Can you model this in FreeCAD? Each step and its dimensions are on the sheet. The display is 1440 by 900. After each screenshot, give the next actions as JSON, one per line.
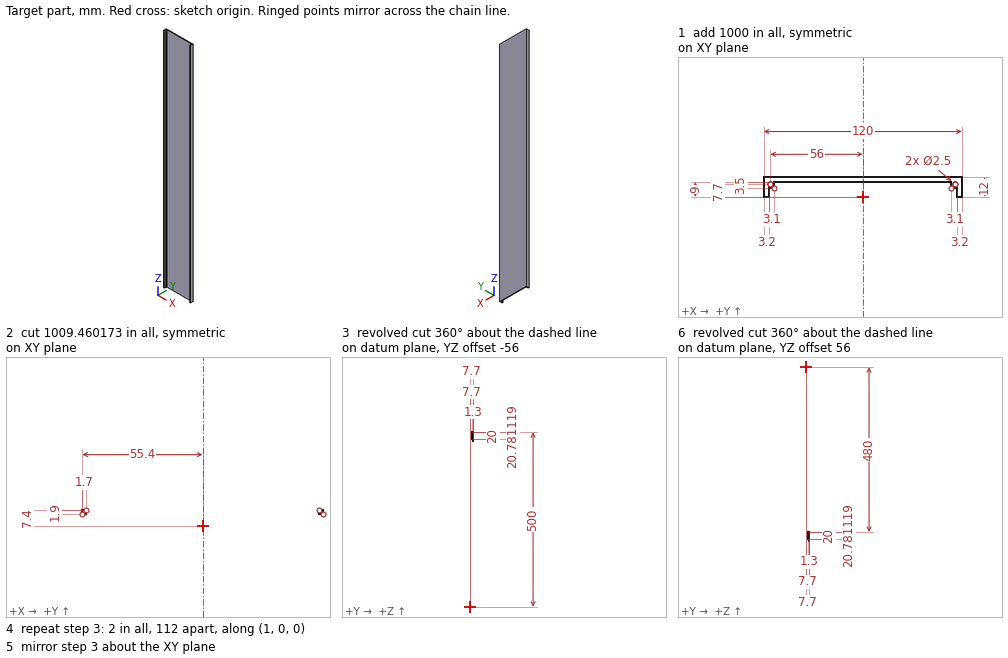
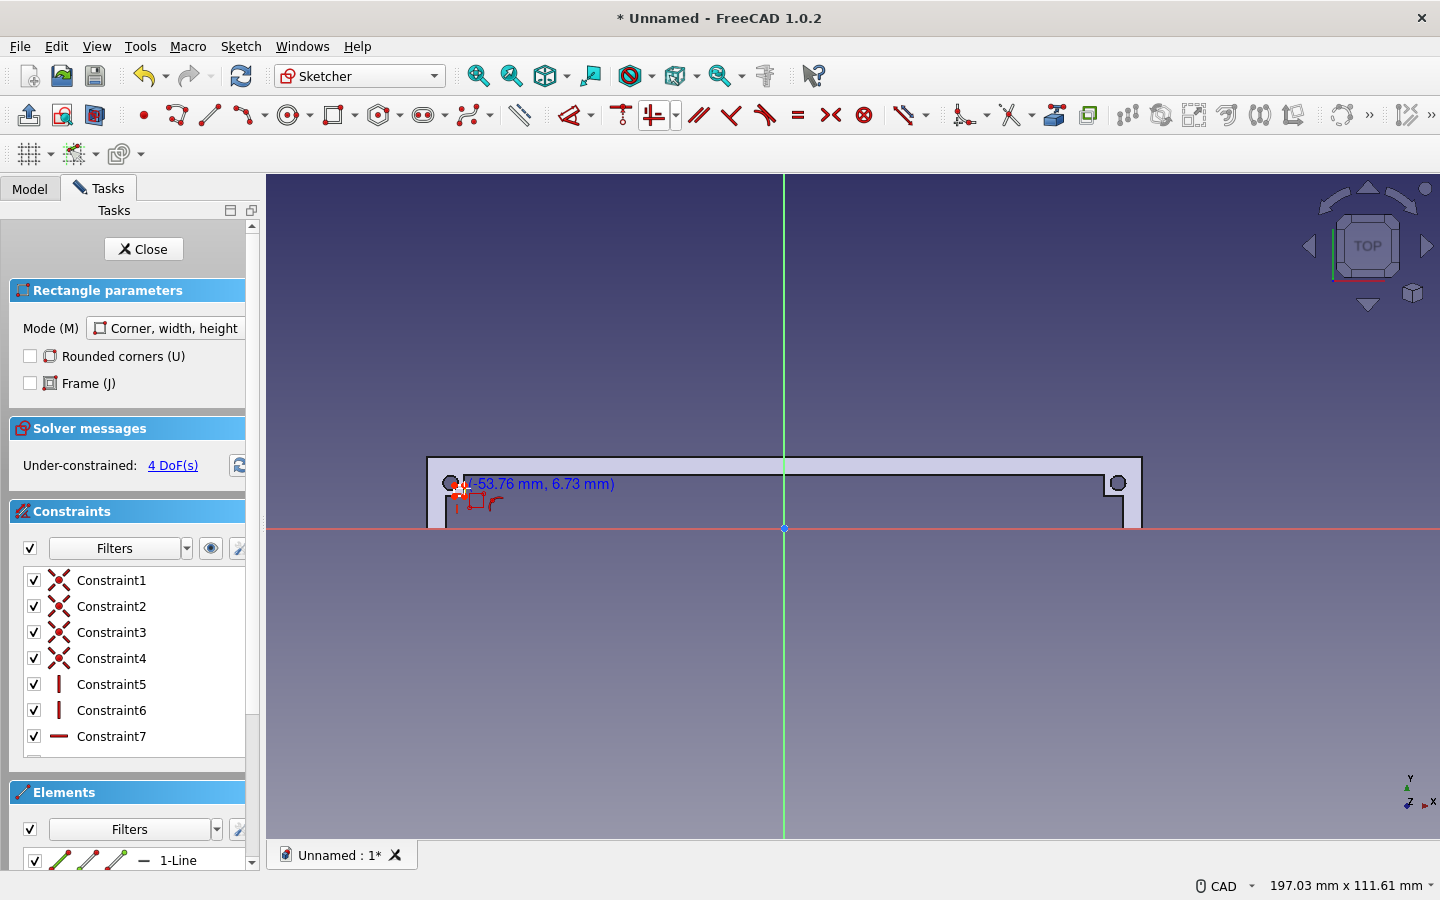
{"action": "scroll", "coordinate": [1104, 485], "scroll_direction": "up", "scroll_amount": 3}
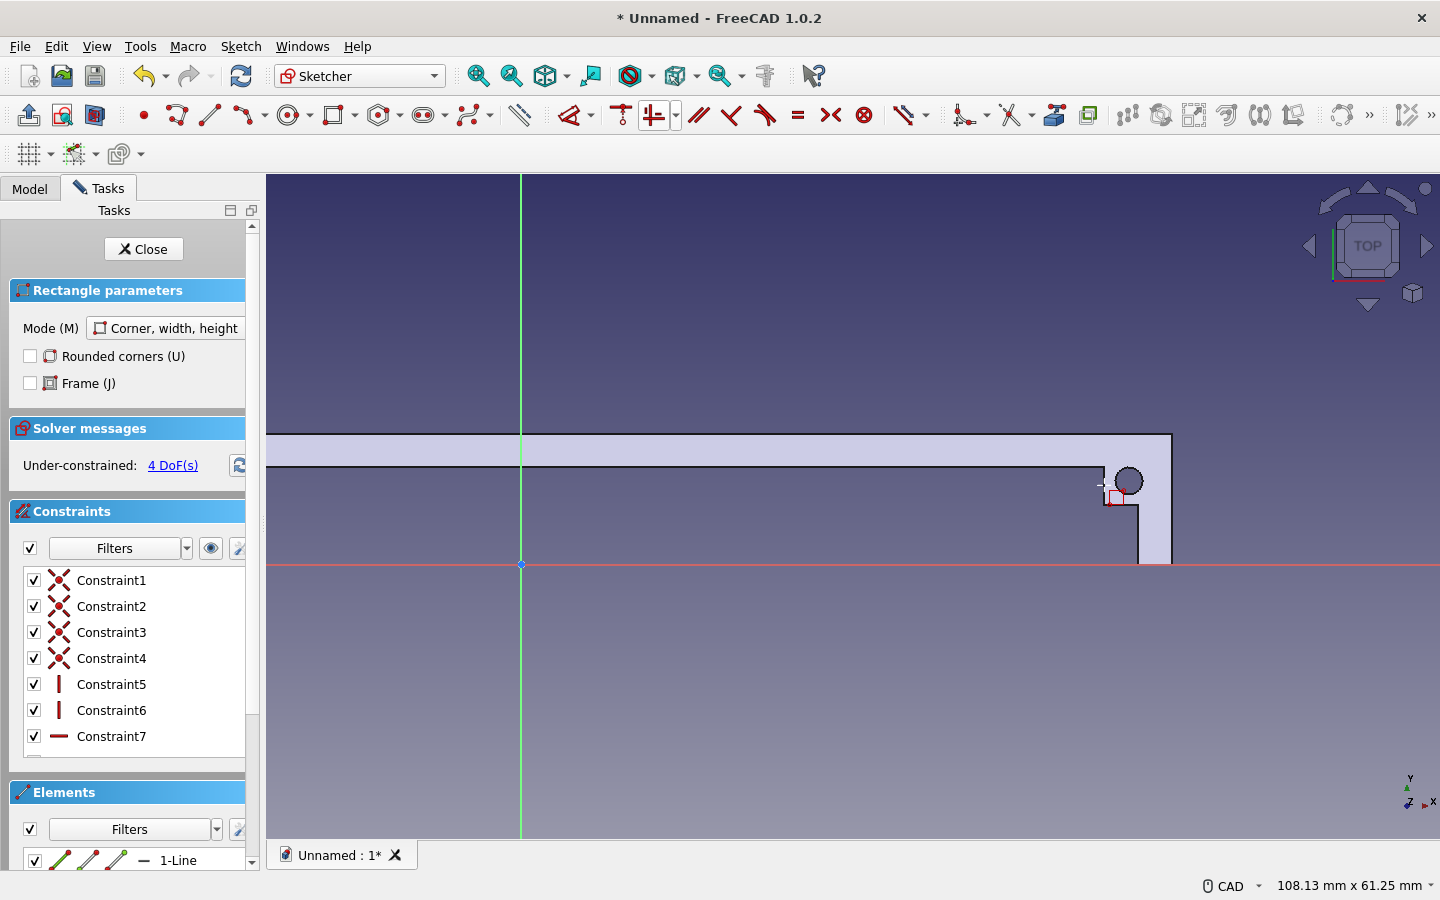
{"action": "left_click", "coordinate": [1104, 484]}
{"action": "left_click", "coordinate": [1122, 505]}
{"action": "key", "text": "Escape"}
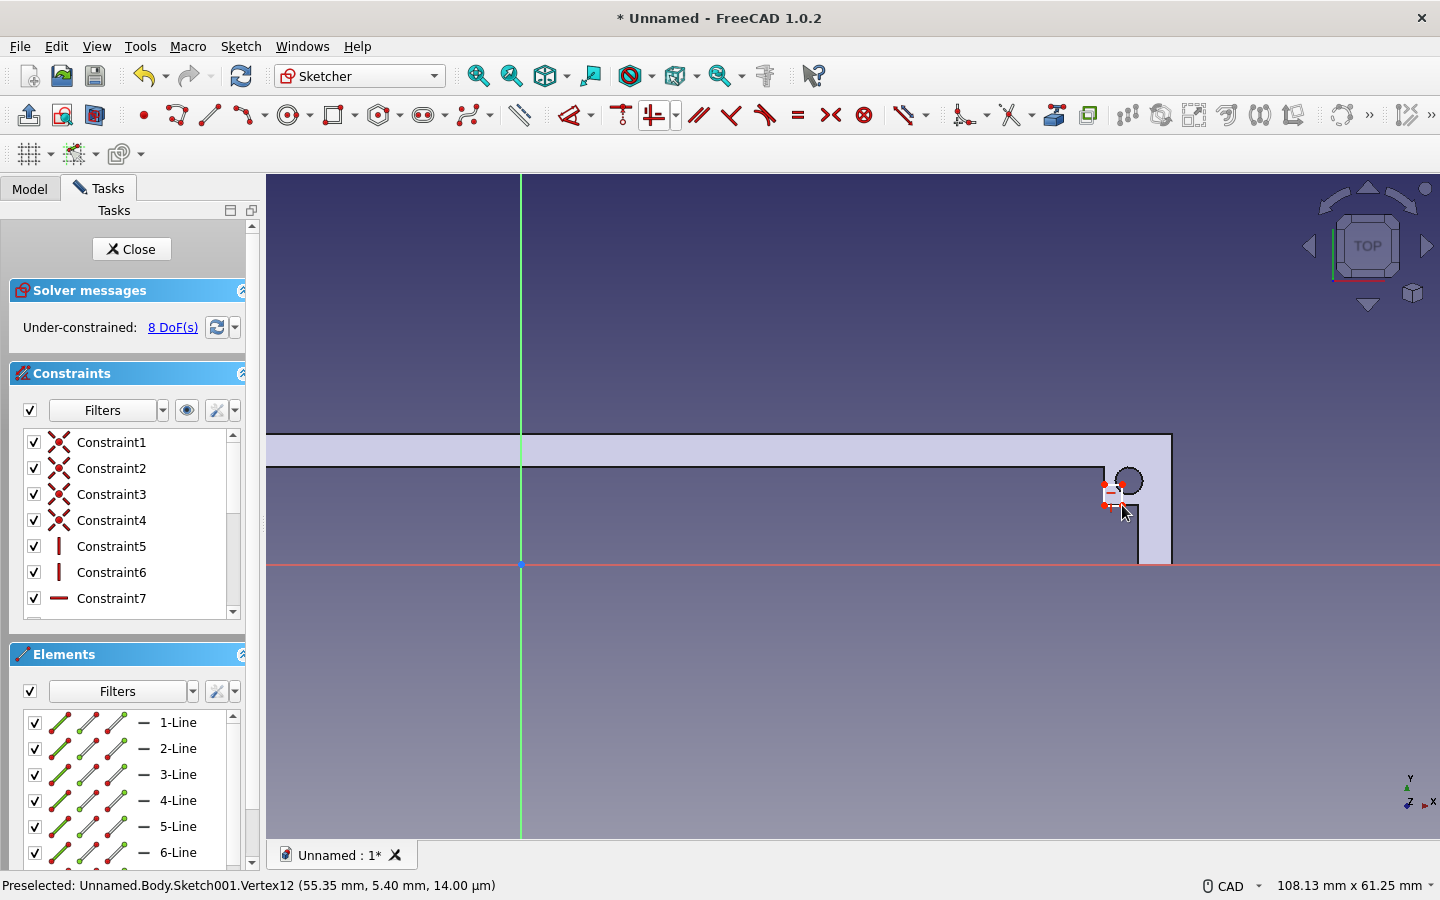
{"action": "scroll", "coordinate": [1105, 485], "scroll_direction": "down", "scroll_amount": 3}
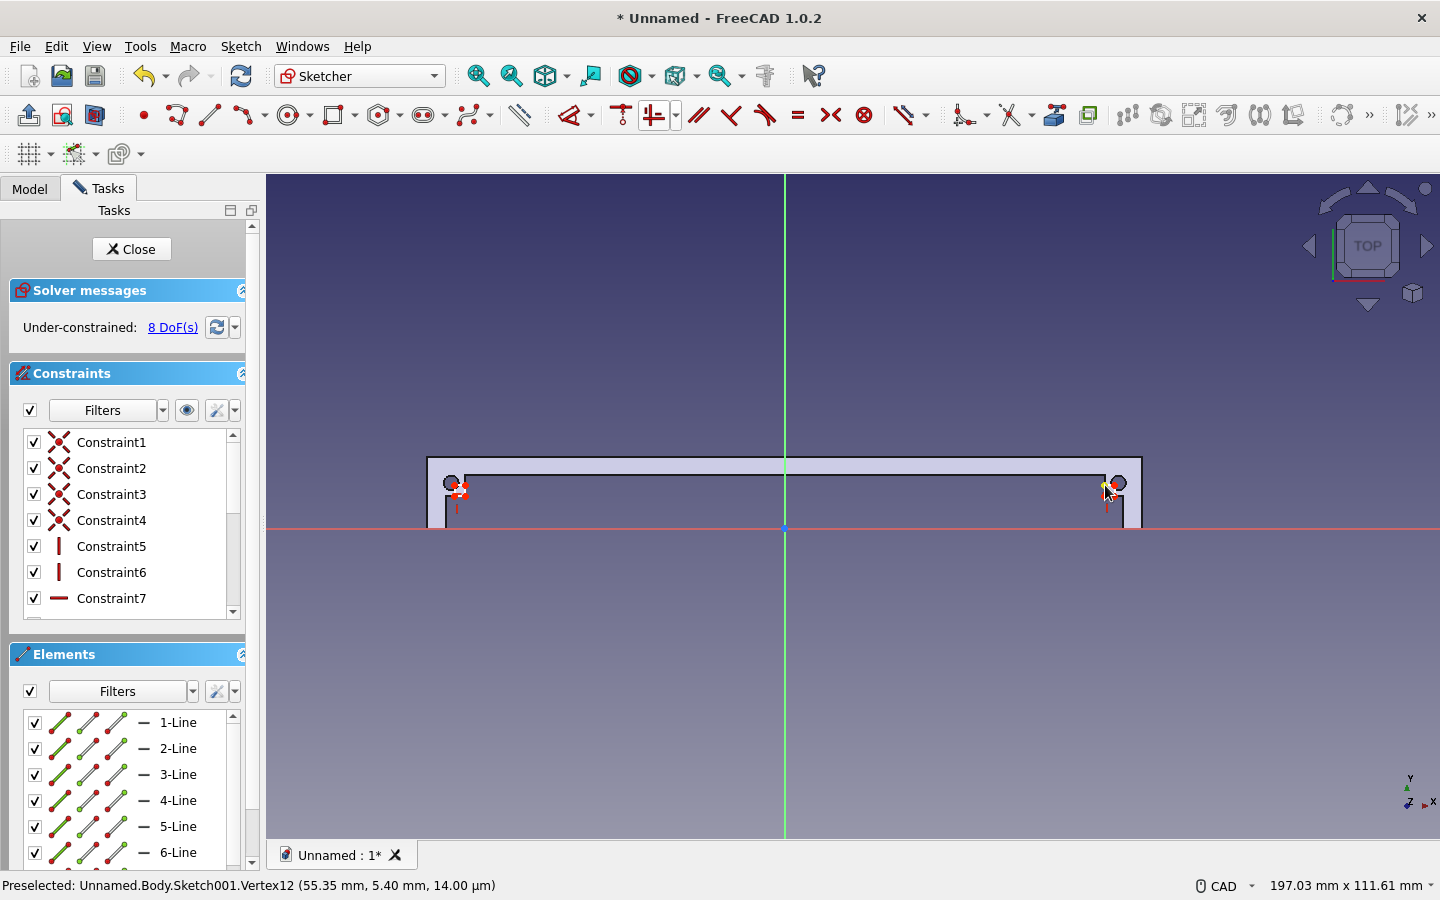
{"action": "left_click", "coordinate": [465, 485]}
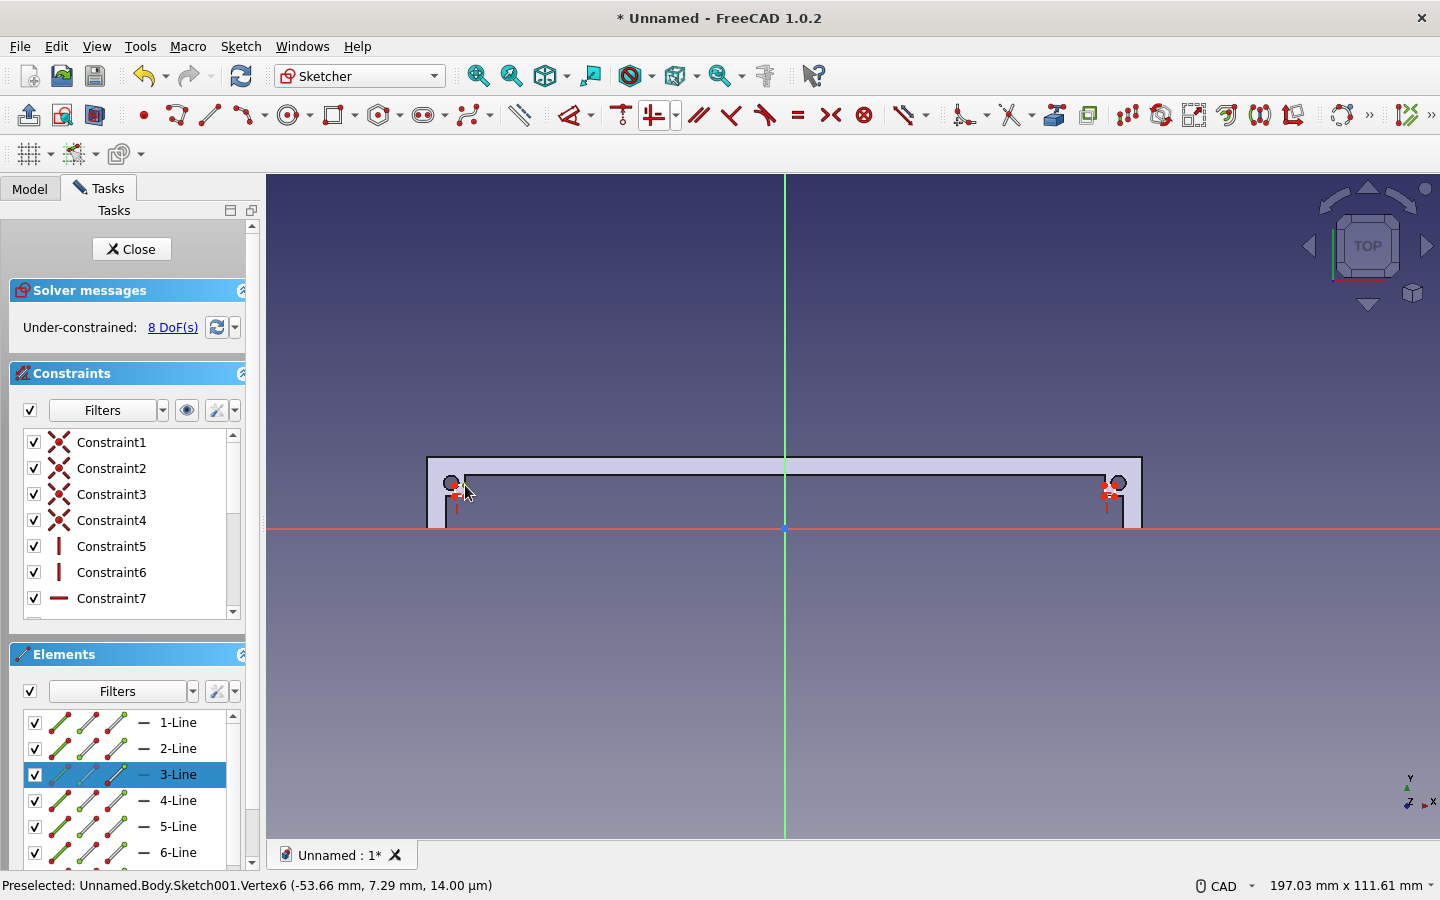
{"action": "scroll", "coordinate": [1105, 485], "scroll_direction": "up", "scroll_amount": 2}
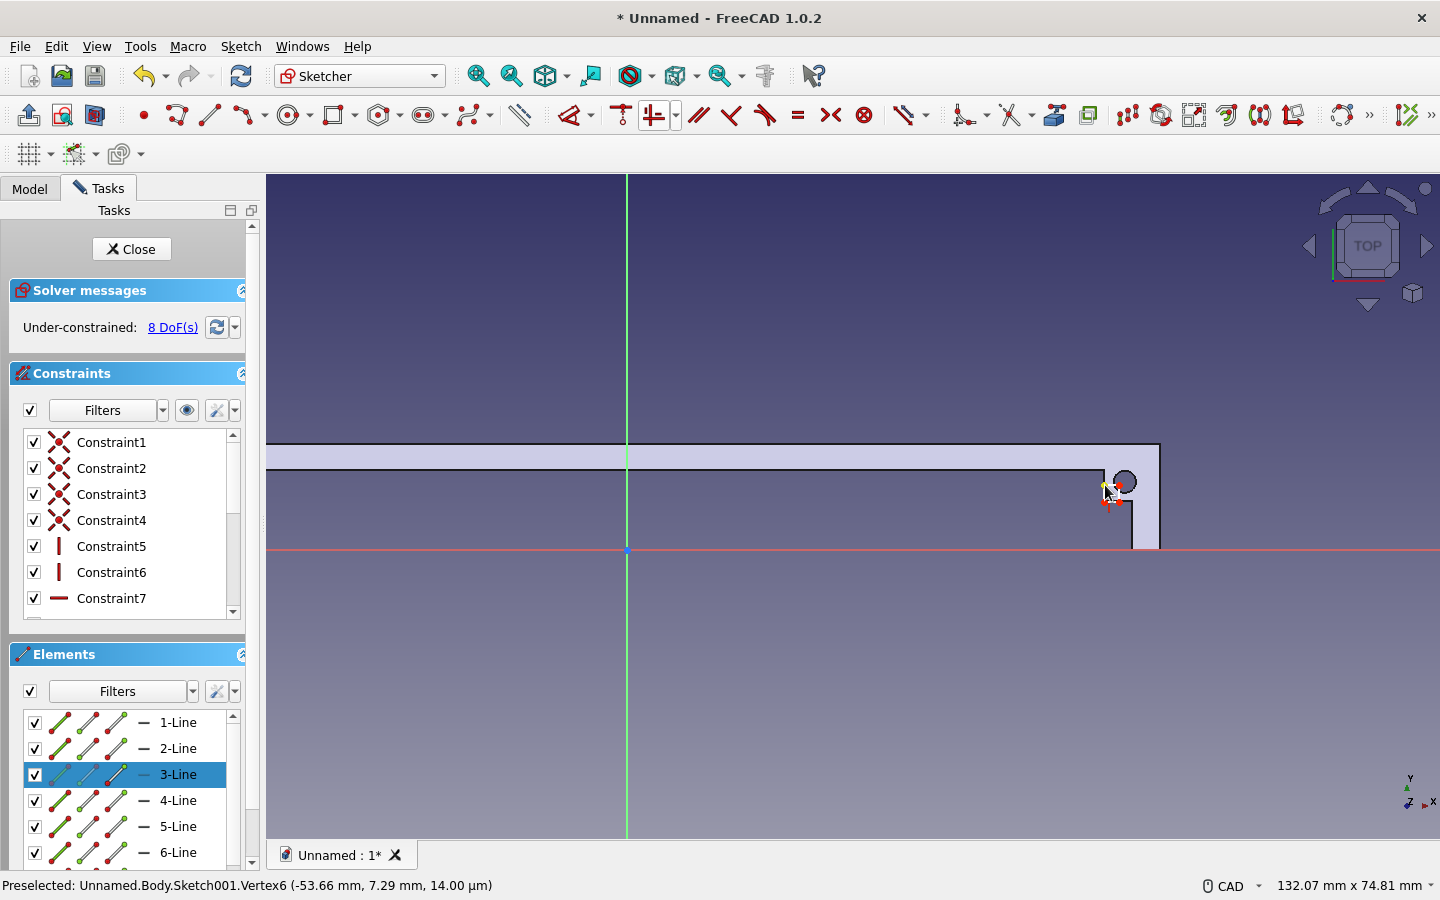
{"action": "left_click", "coordinate": [1104, 485]}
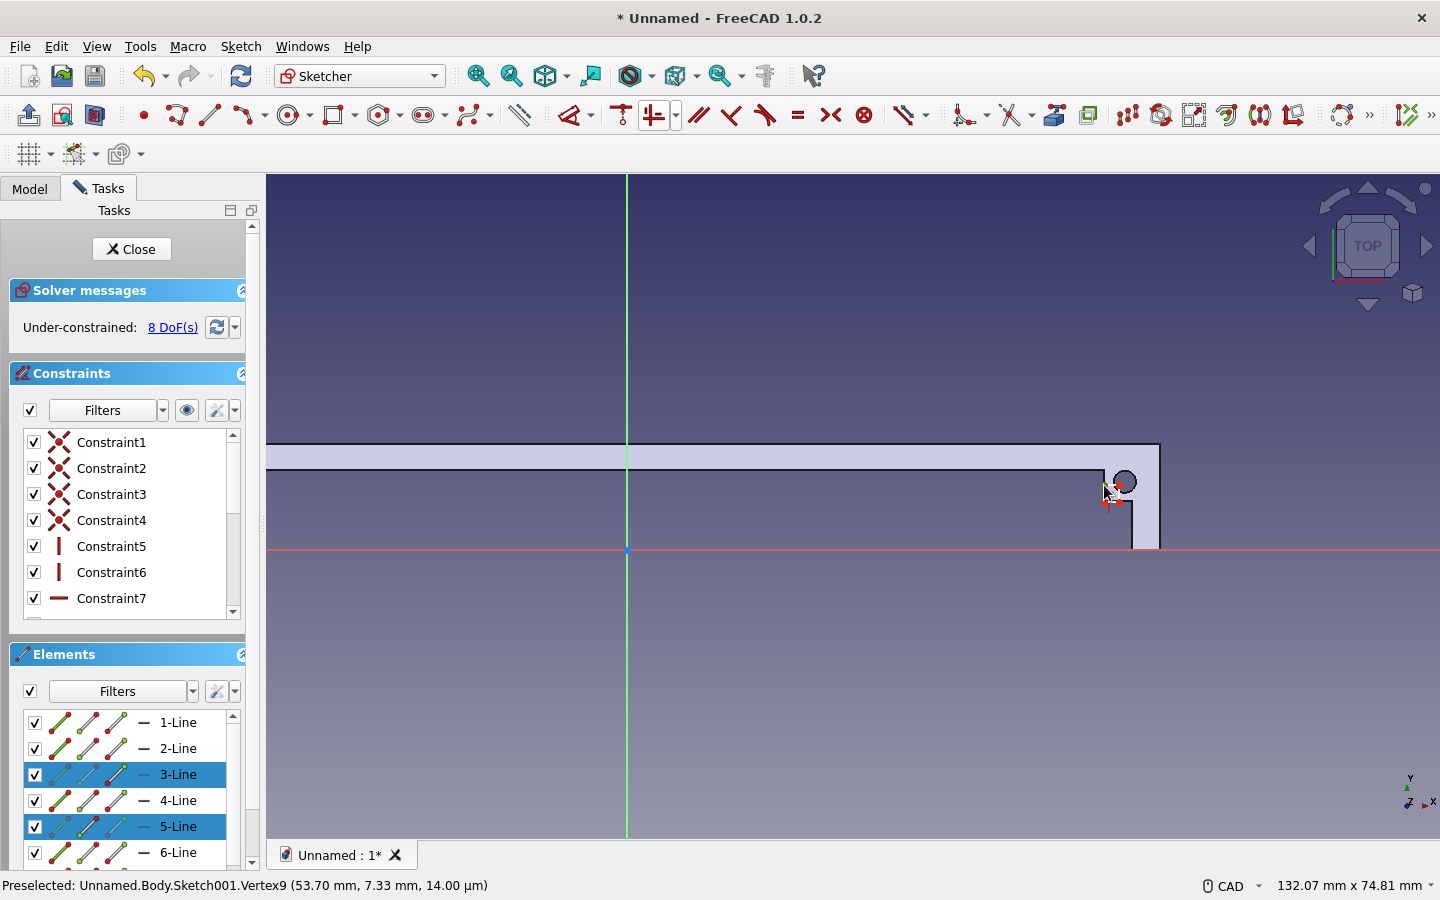
{"action": "left_click", "coordinate": [627, 768]}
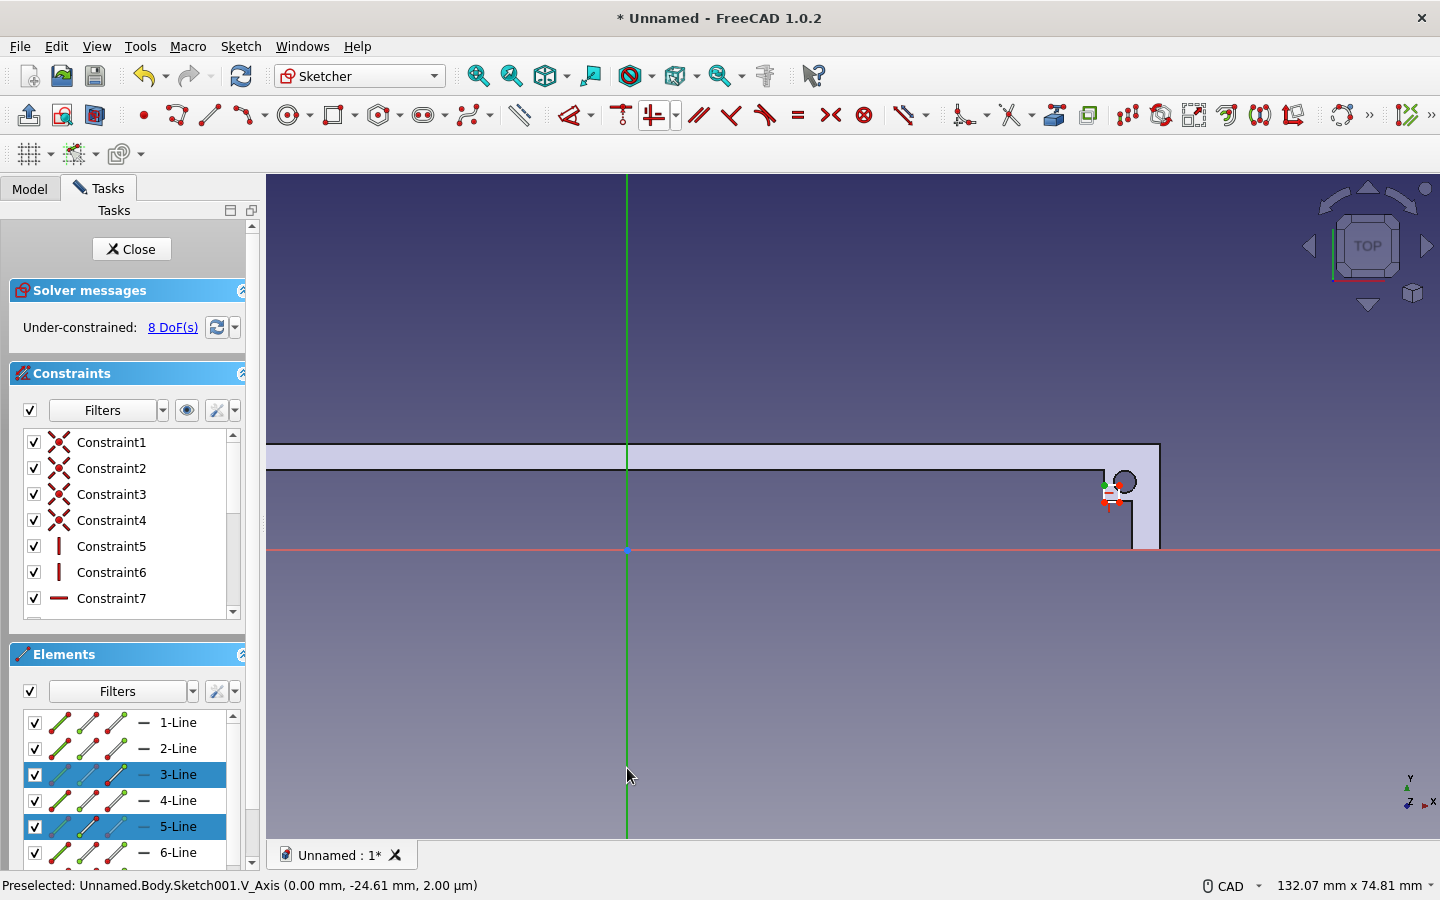
{"action": "key", "text": "s"}